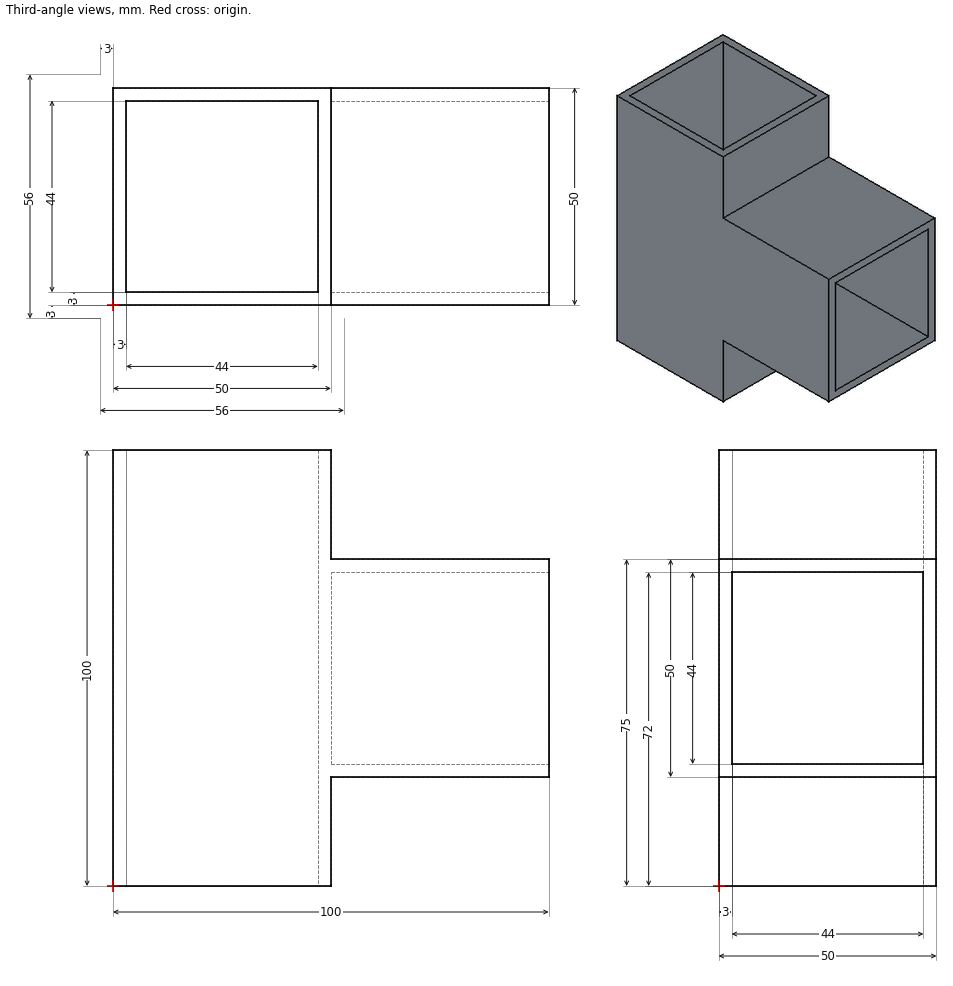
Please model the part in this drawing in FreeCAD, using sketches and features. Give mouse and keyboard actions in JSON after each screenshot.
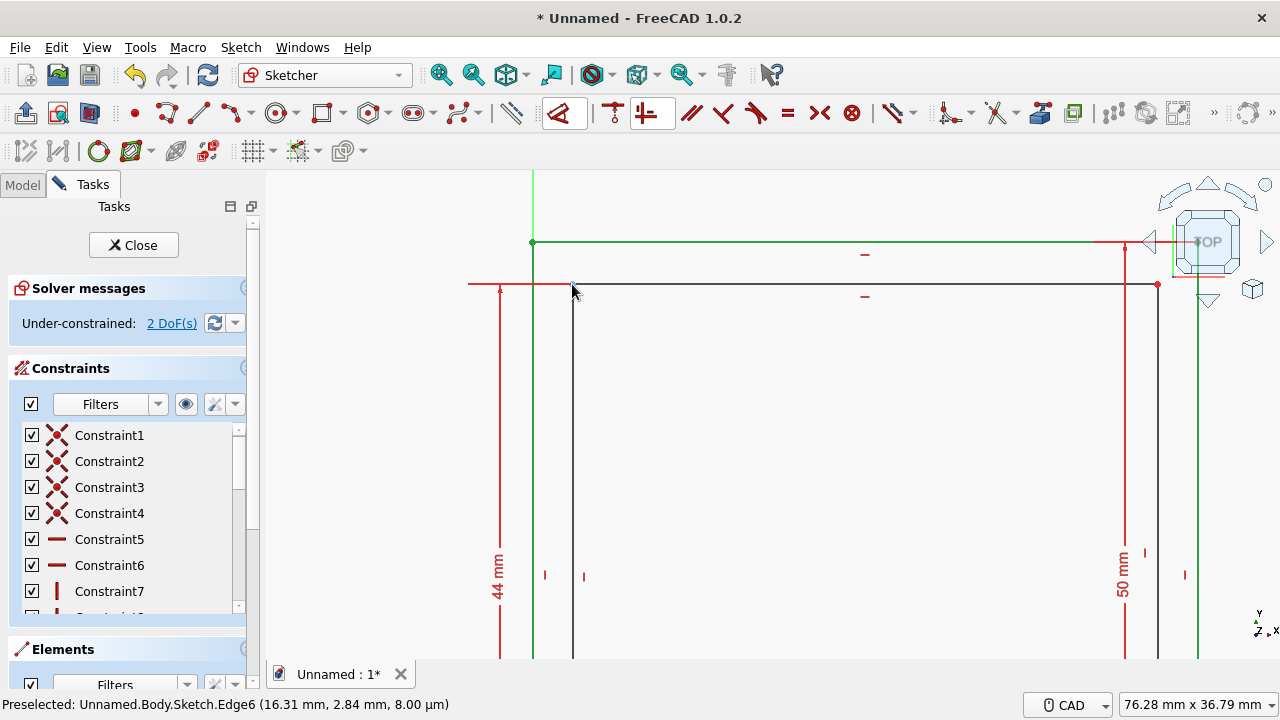
{"action": "left_click", "coordinate": [573, 284]}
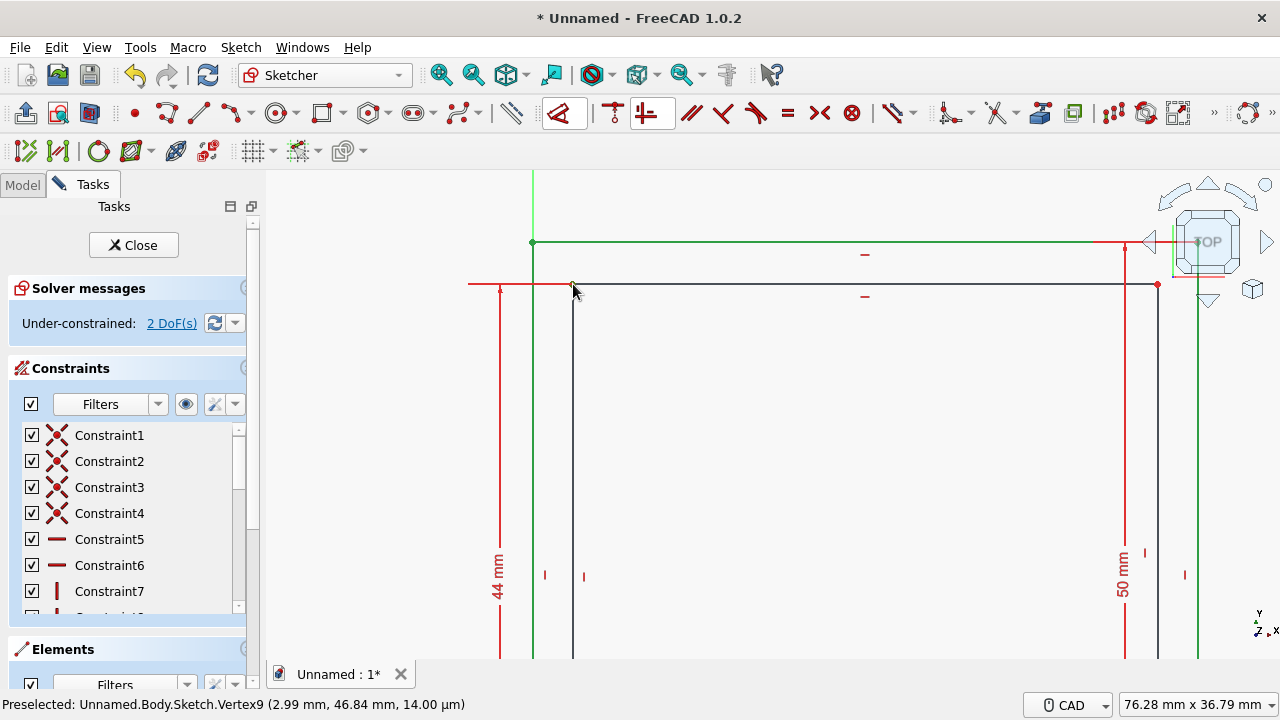
{"action": "left_click", "coordinate": [582, 114]}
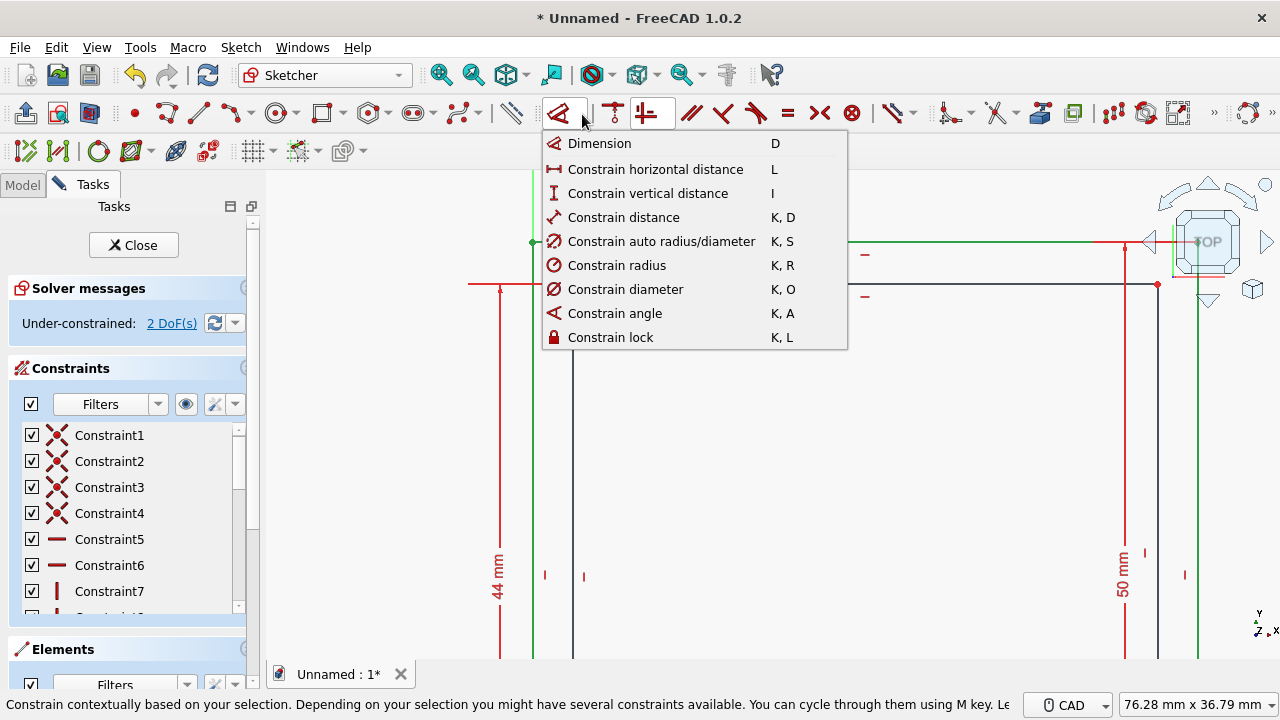
{"action": "left_click", "coordinate": [695, 169]}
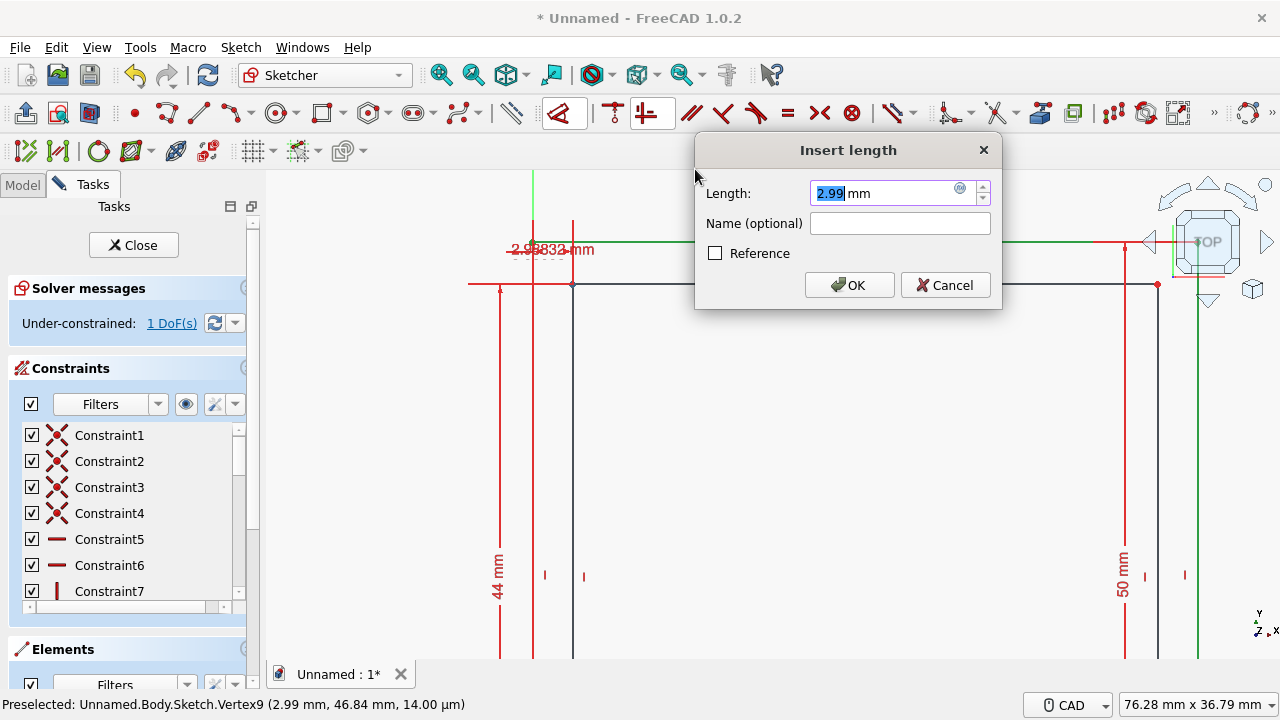
{"action": "type", "text": "3"}
{"action": "key", "text": "Return"}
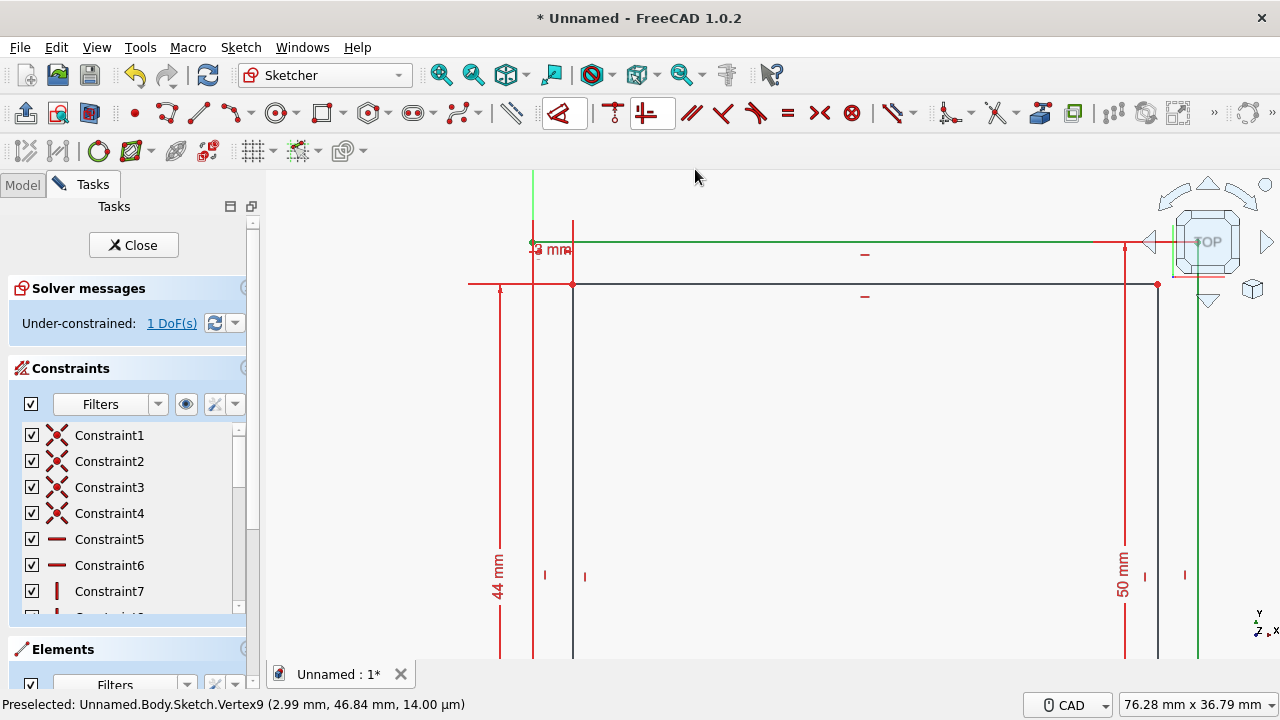
{"action": "scroll", "coordinate": [573, 284], "scroll_direction": "down", "scroll_amount": 4}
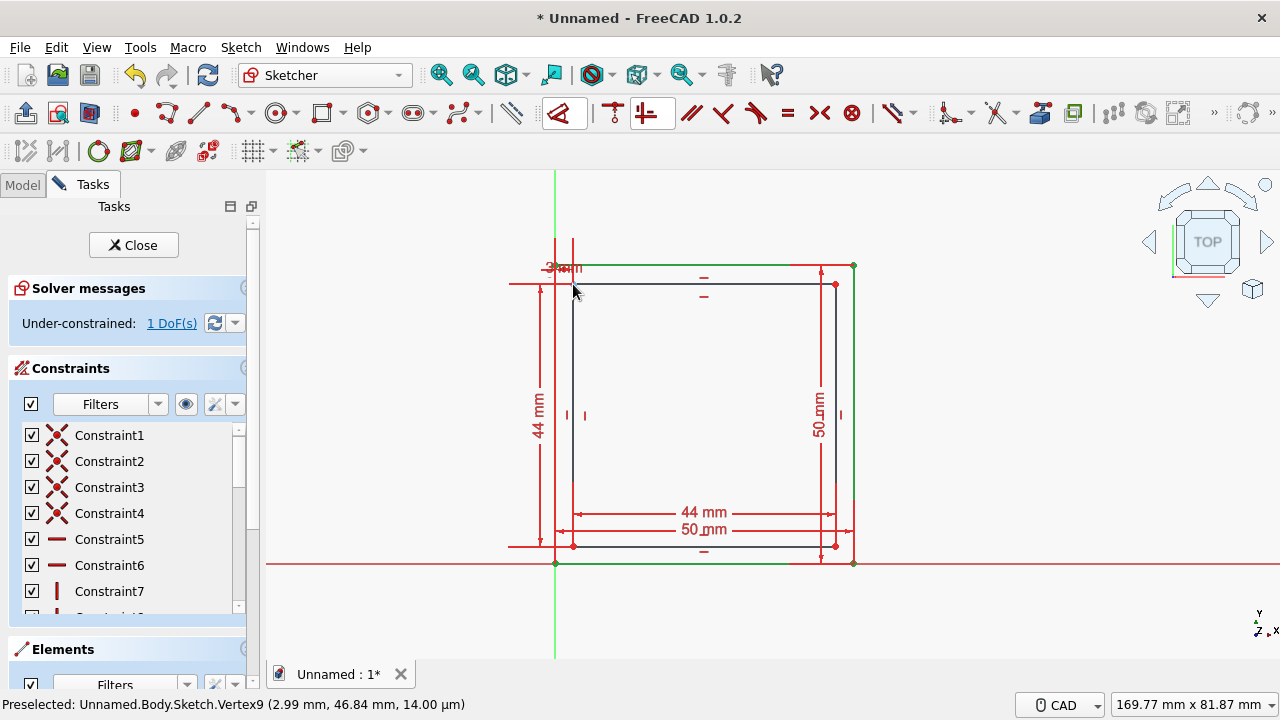
{"action": "scroll", "coordinate": [573, 547], "scroll_direction": "up", "scroll_amount": 4}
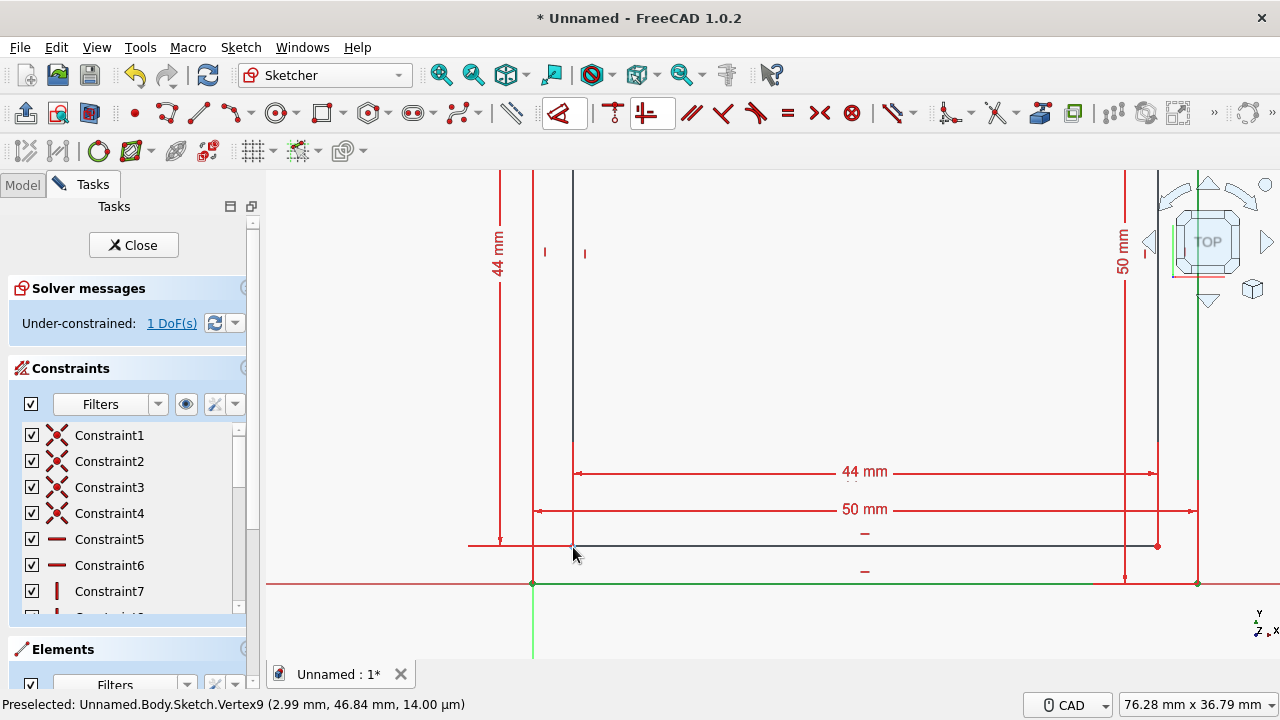
{"action": "left_click", "coordinate": [573, 546]}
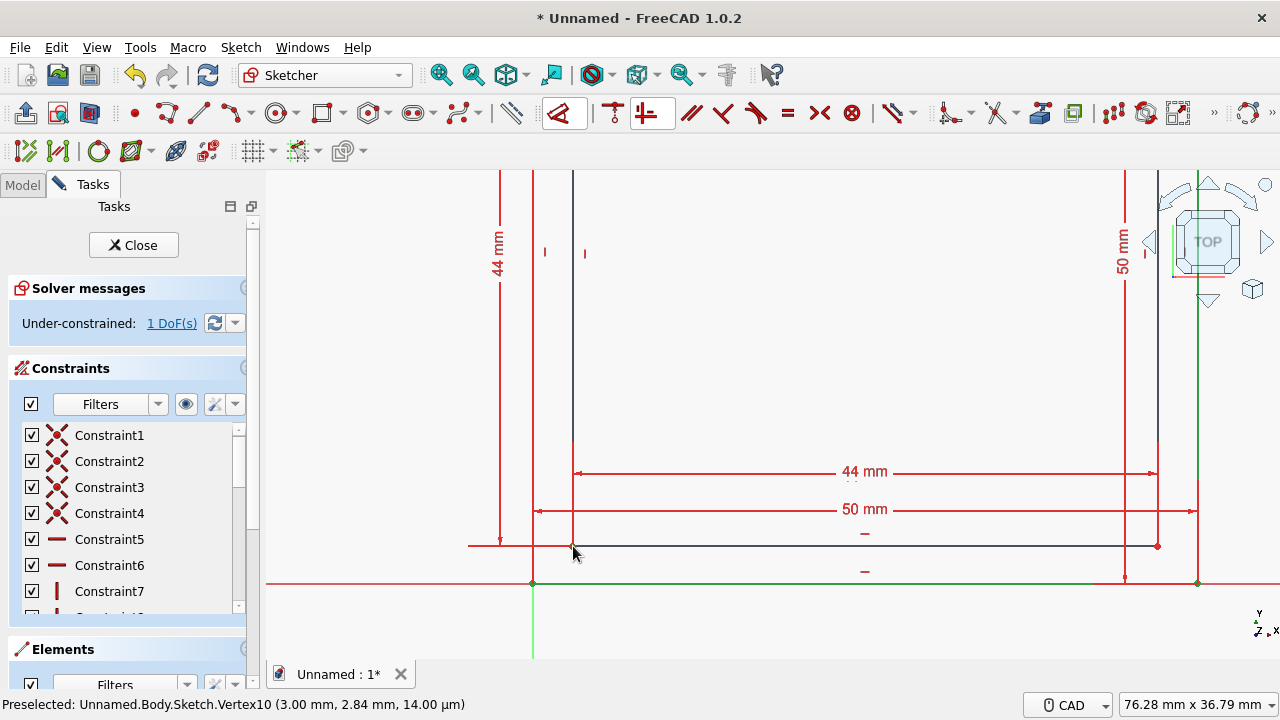
{"action": "key", "text": "i"}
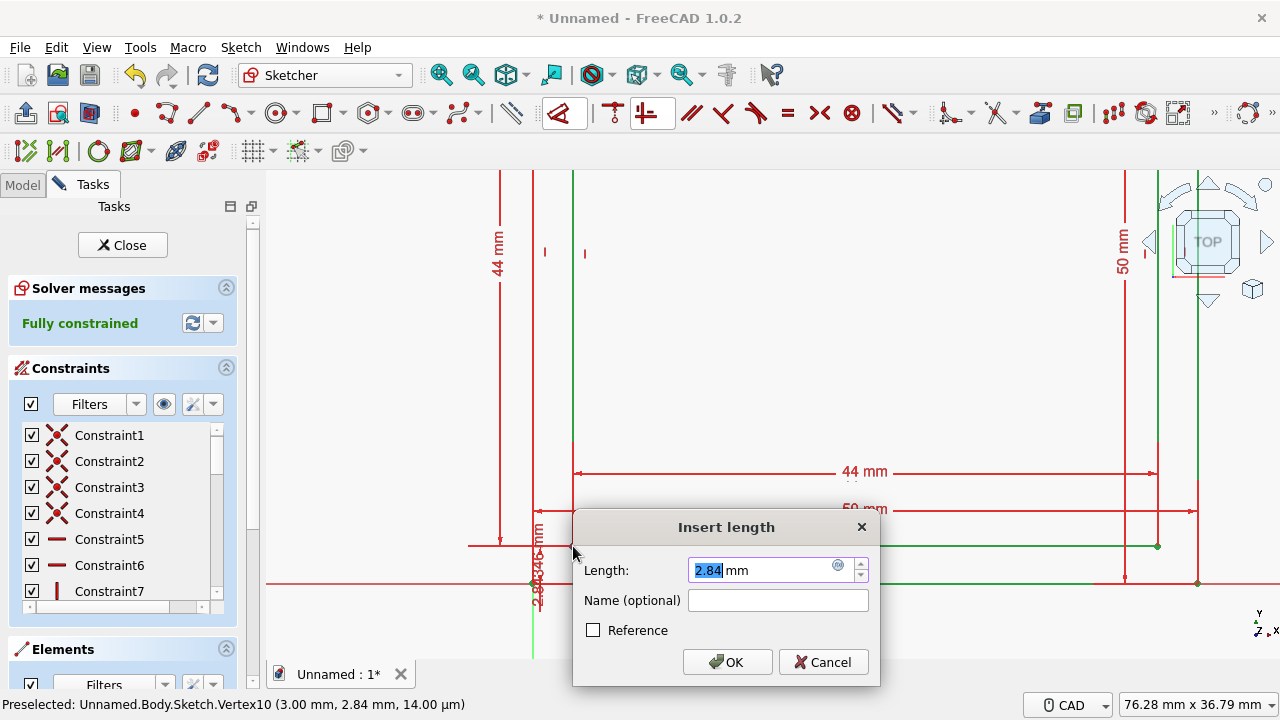
{"action": "type", "text": "3"}
{"action": "key", "text": "Return"}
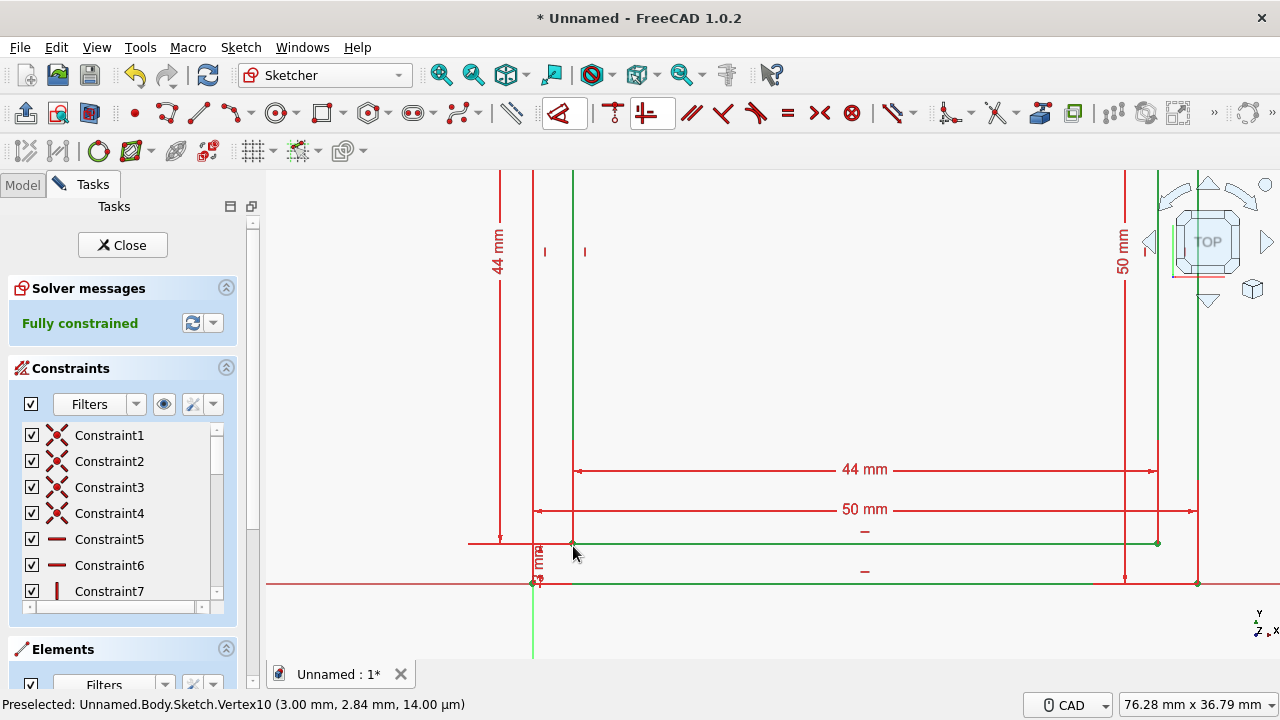
{"action": "left_click", "coordinate": [123, 245]}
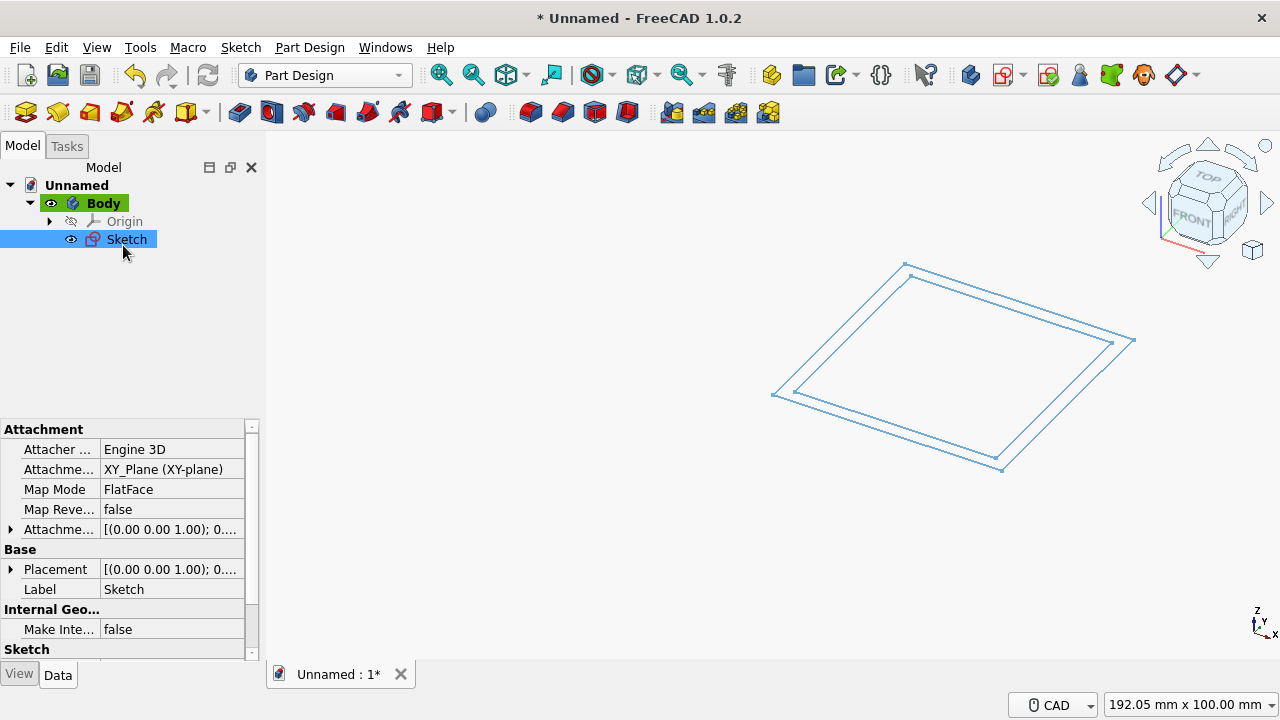
{"action": "left_click", "coordinate": [26, 112]}